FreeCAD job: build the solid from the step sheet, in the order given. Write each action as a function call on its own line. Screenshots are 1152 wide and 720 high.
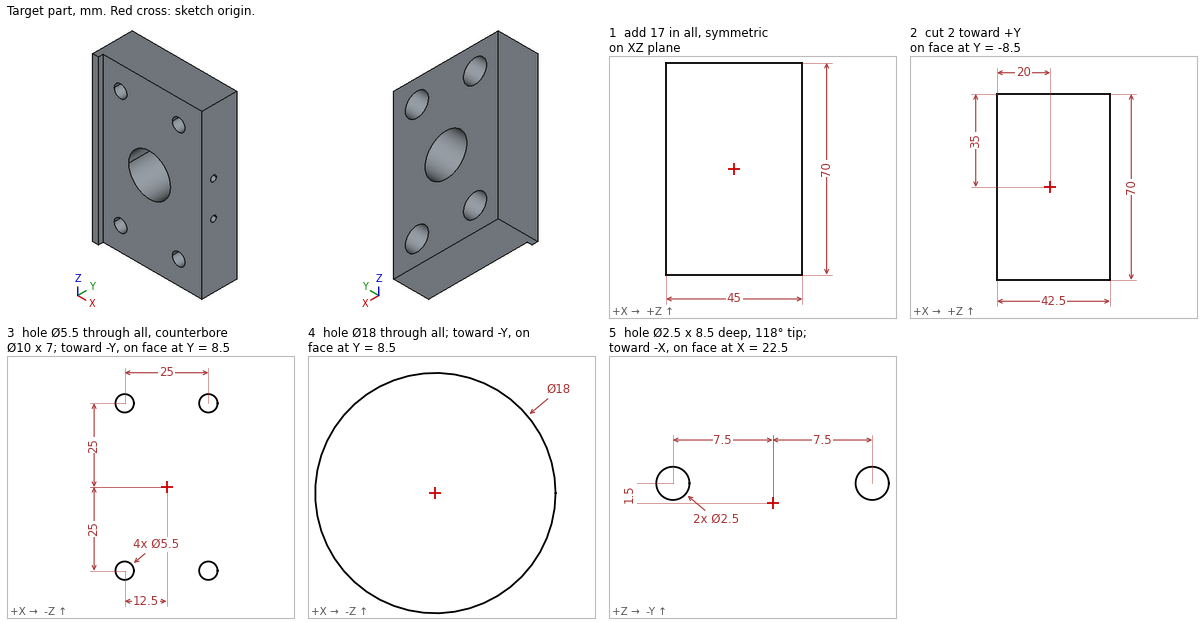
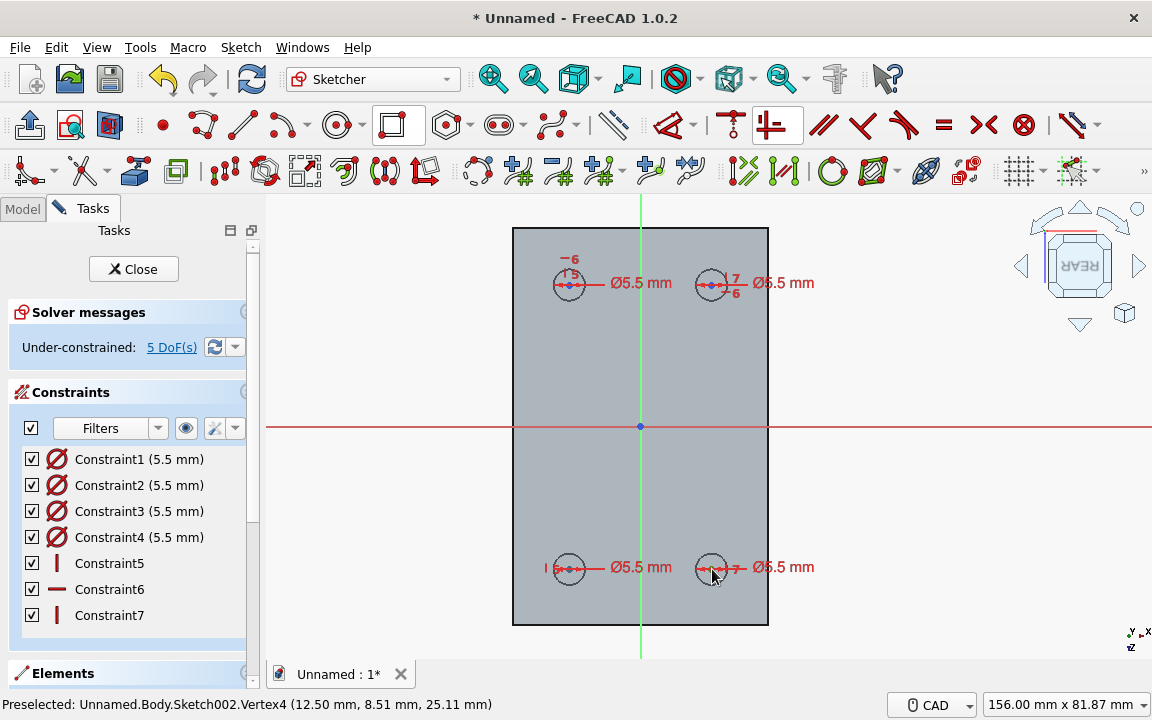
click(798, 126)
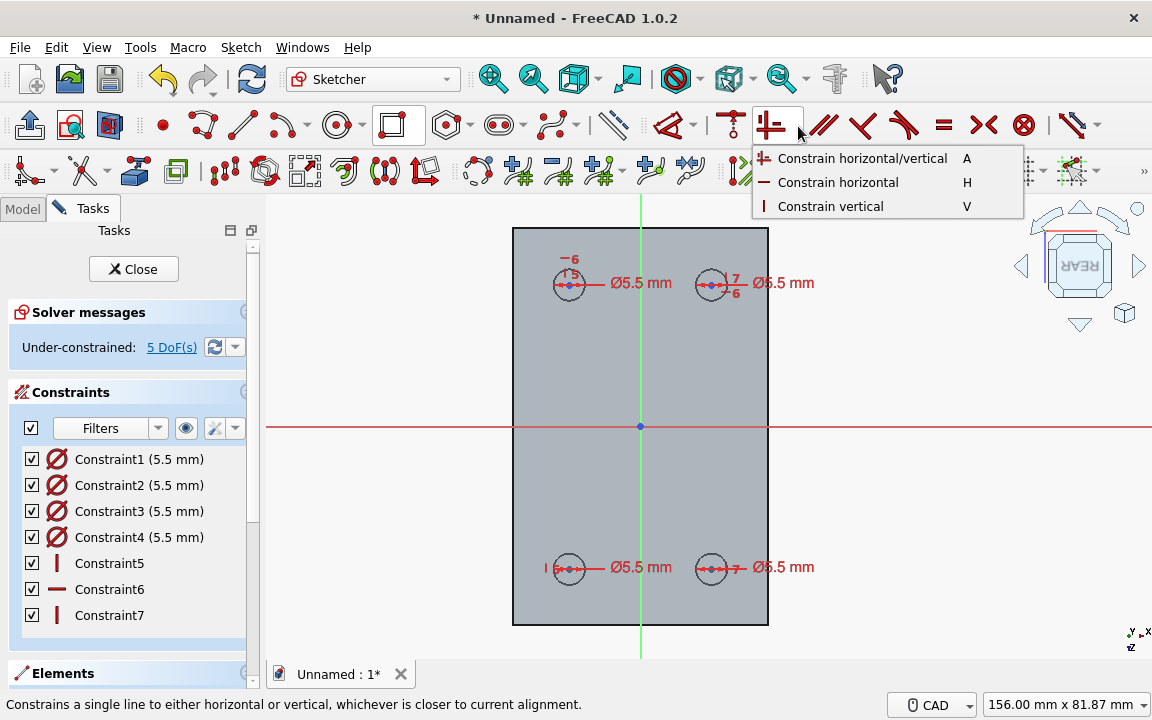
click(888, 182)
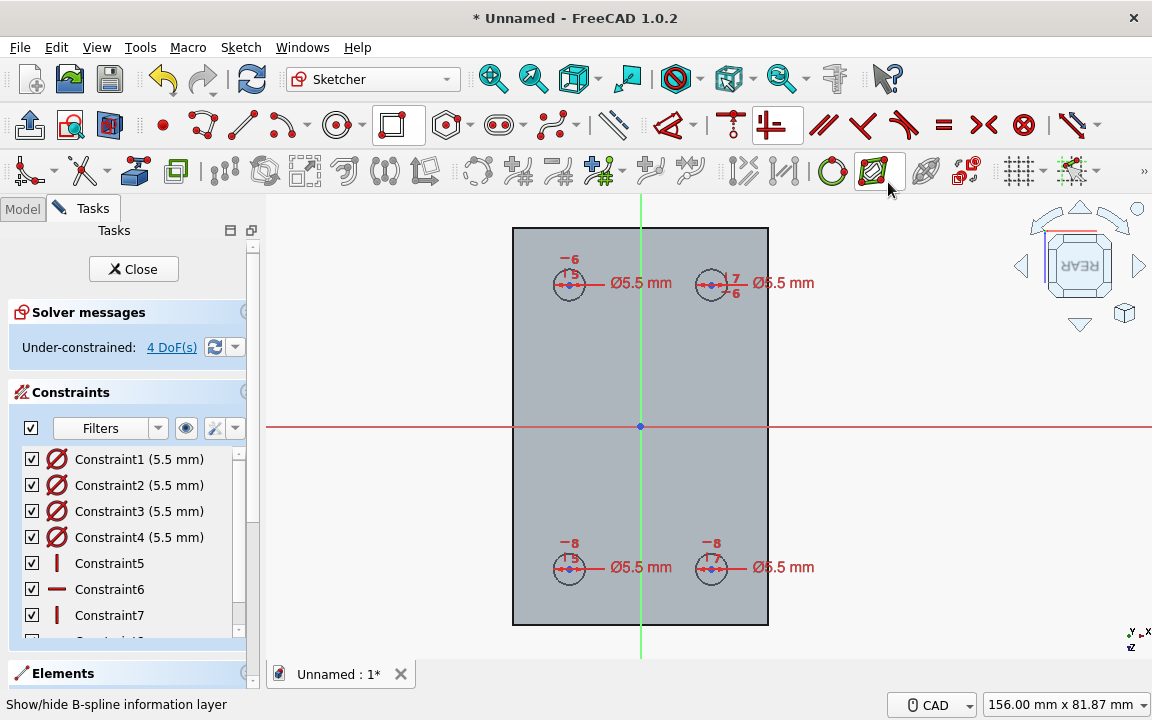
click(668, 126)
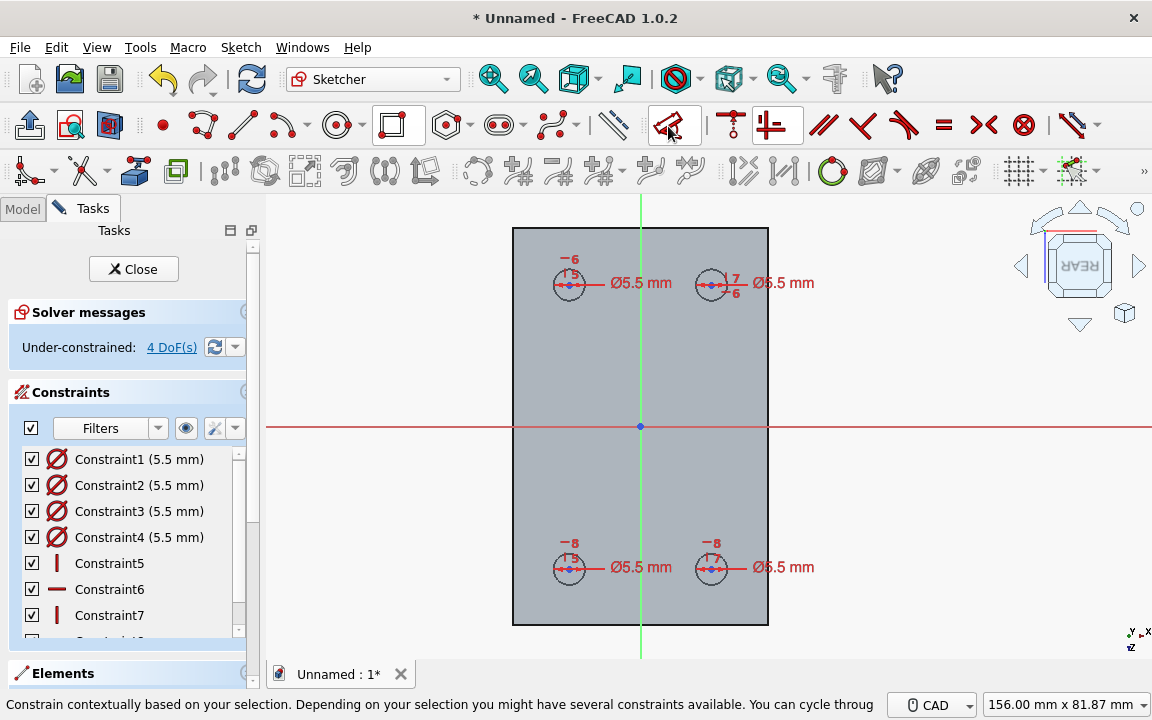
click(569, 569)
click(535, 498)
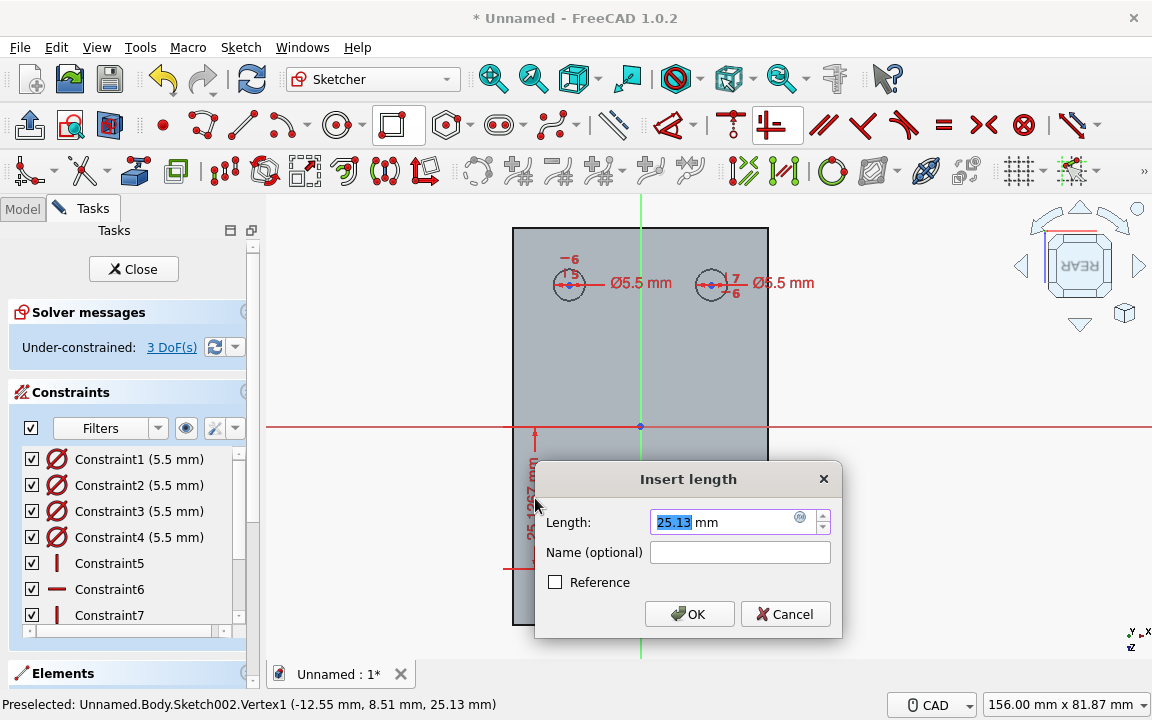
text(25)
key(Return)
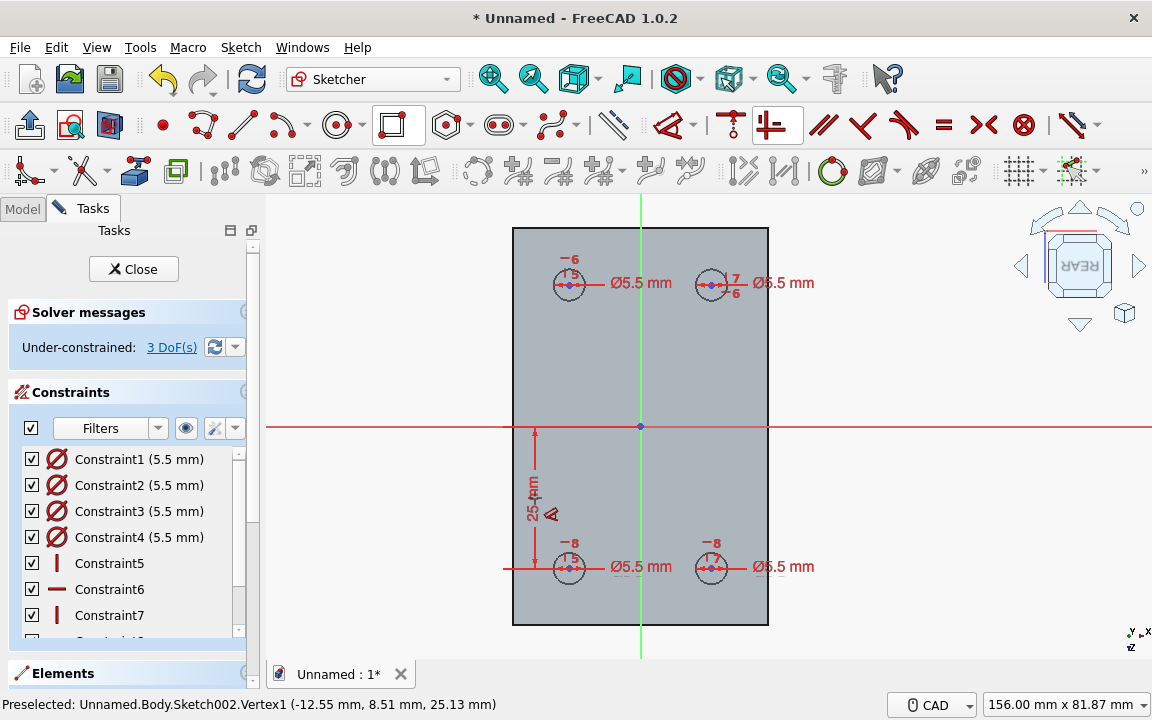
click(569, 285)
click(535, 356)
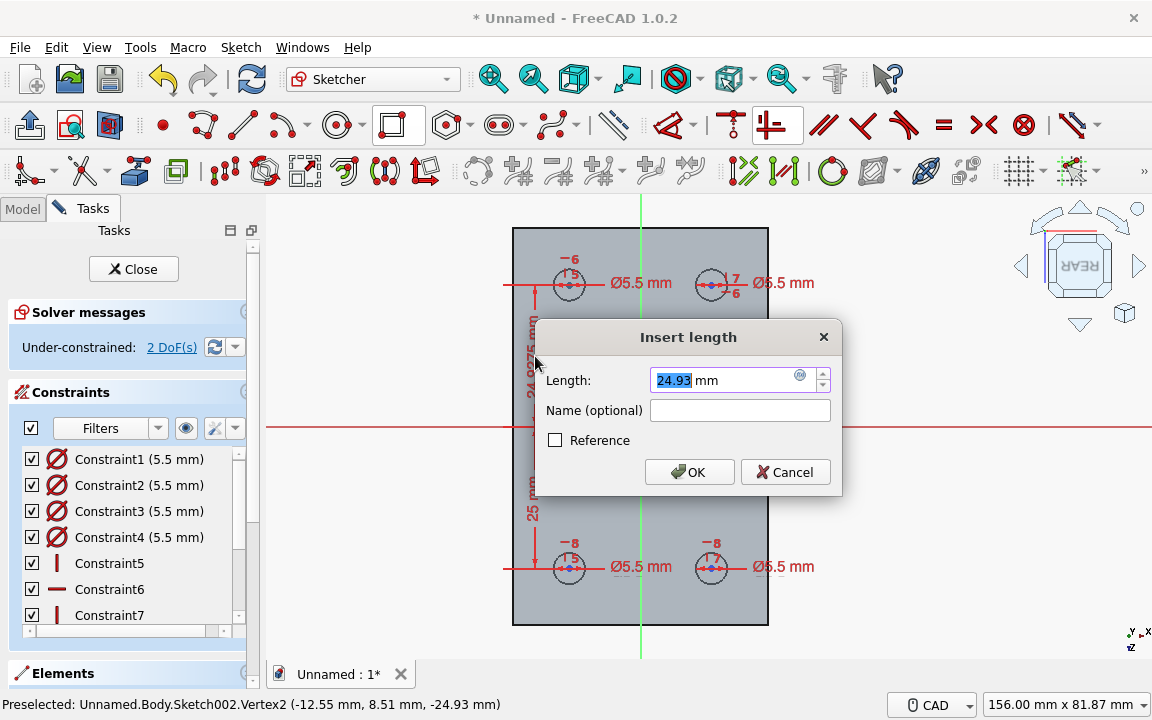
text(25)
key(Return)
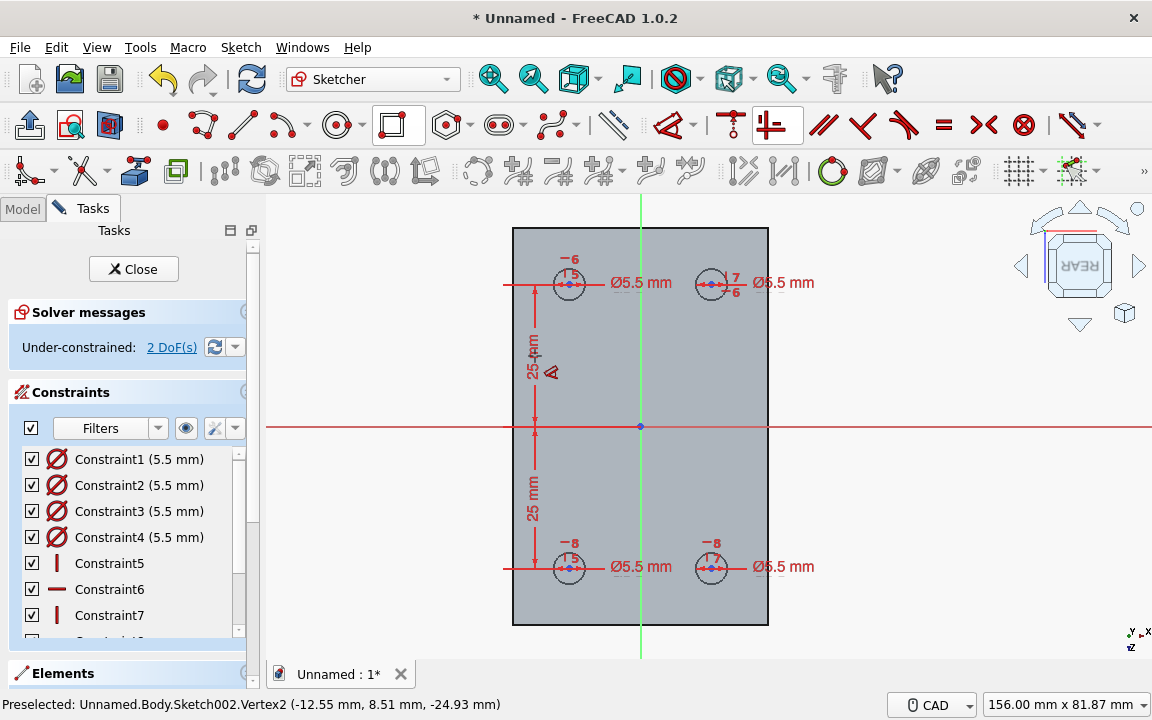
click(569, 285)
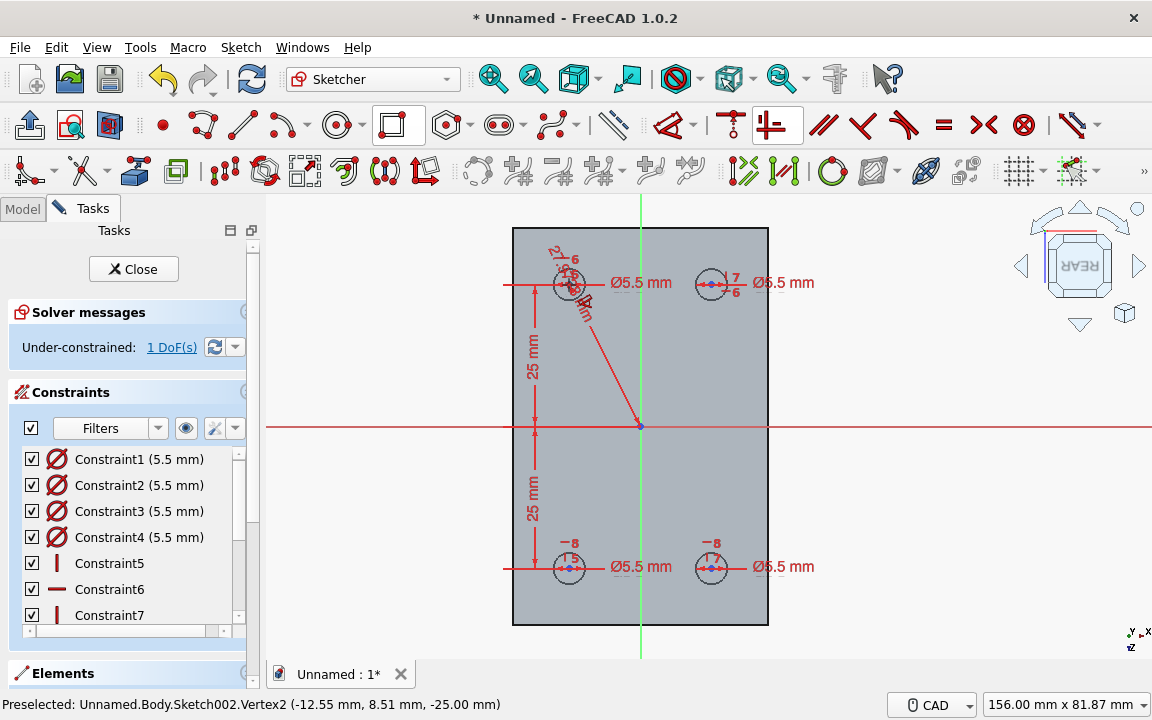
click(712, 285)
click(608, 251)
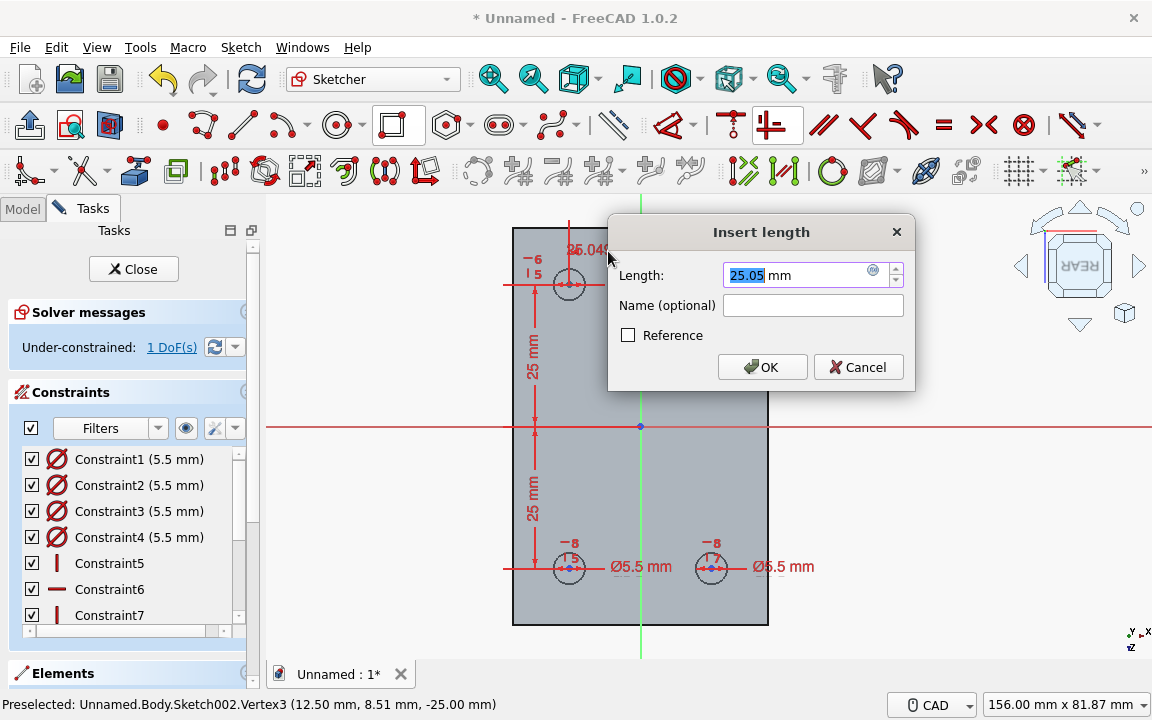
text(25)
key(Return)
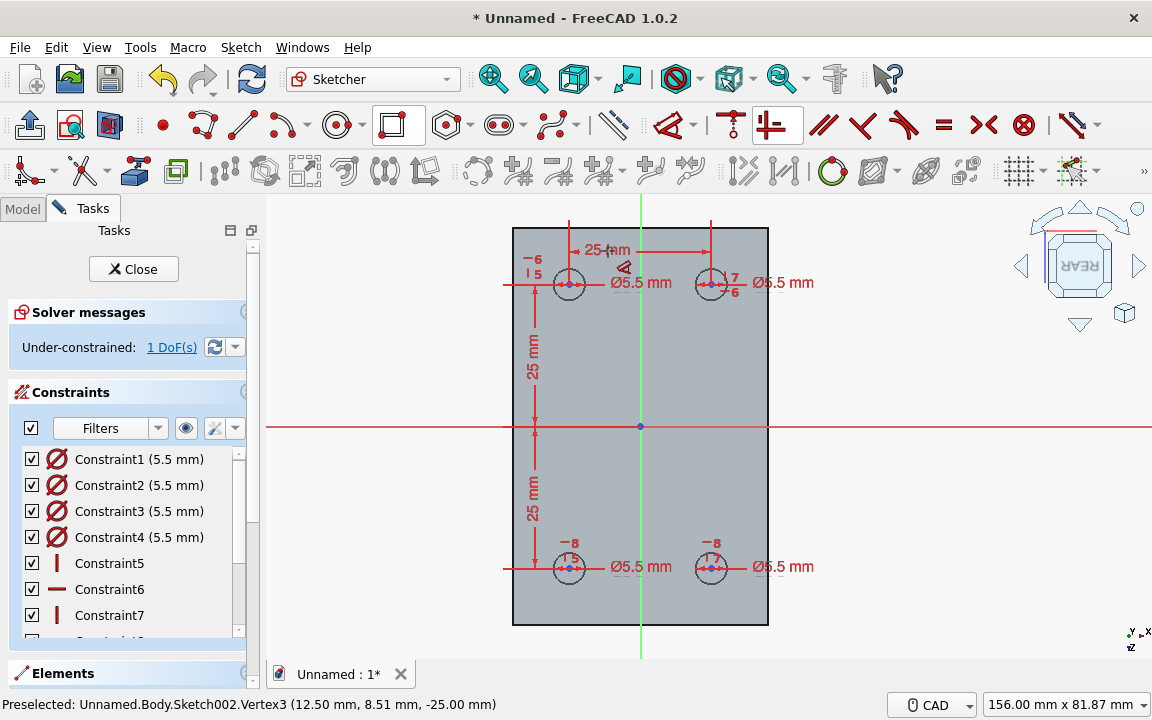
click(569, 569)
click(605, 603)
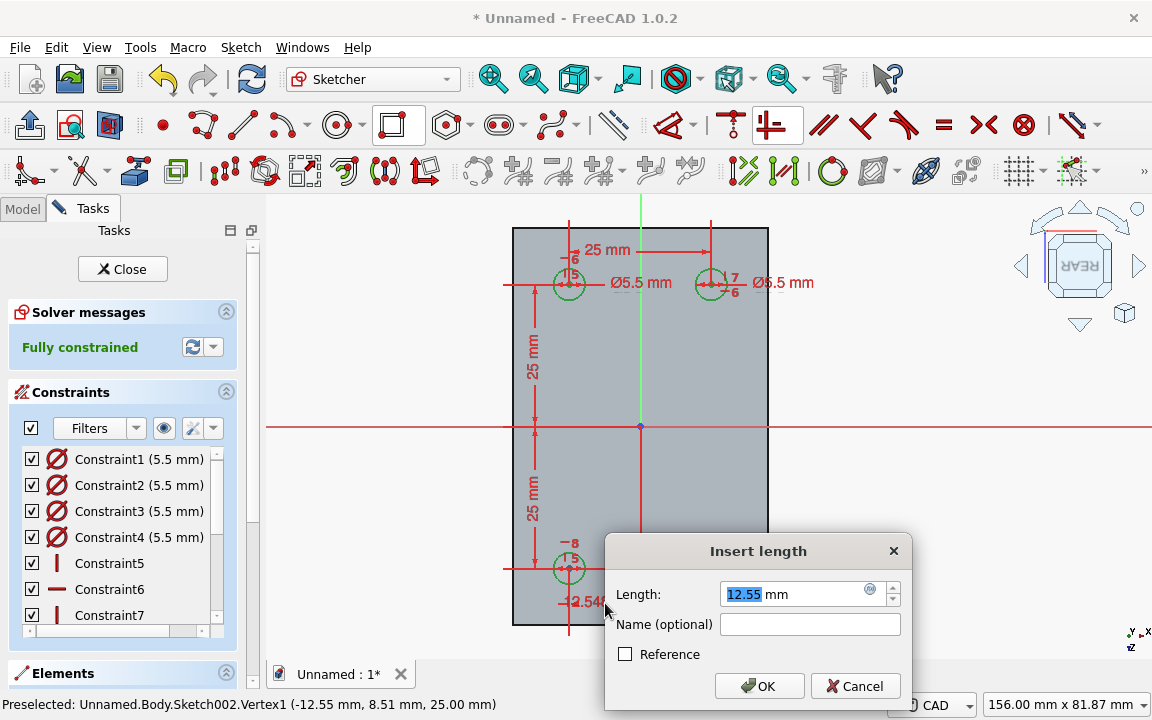
text(12.5)
key(Return)
key(Escape)